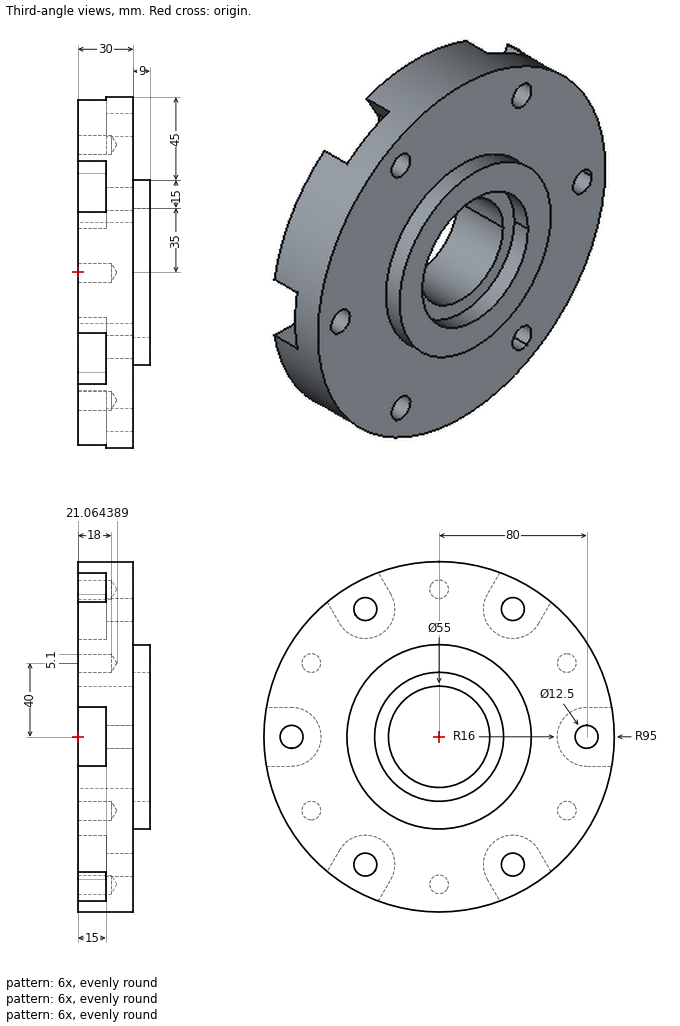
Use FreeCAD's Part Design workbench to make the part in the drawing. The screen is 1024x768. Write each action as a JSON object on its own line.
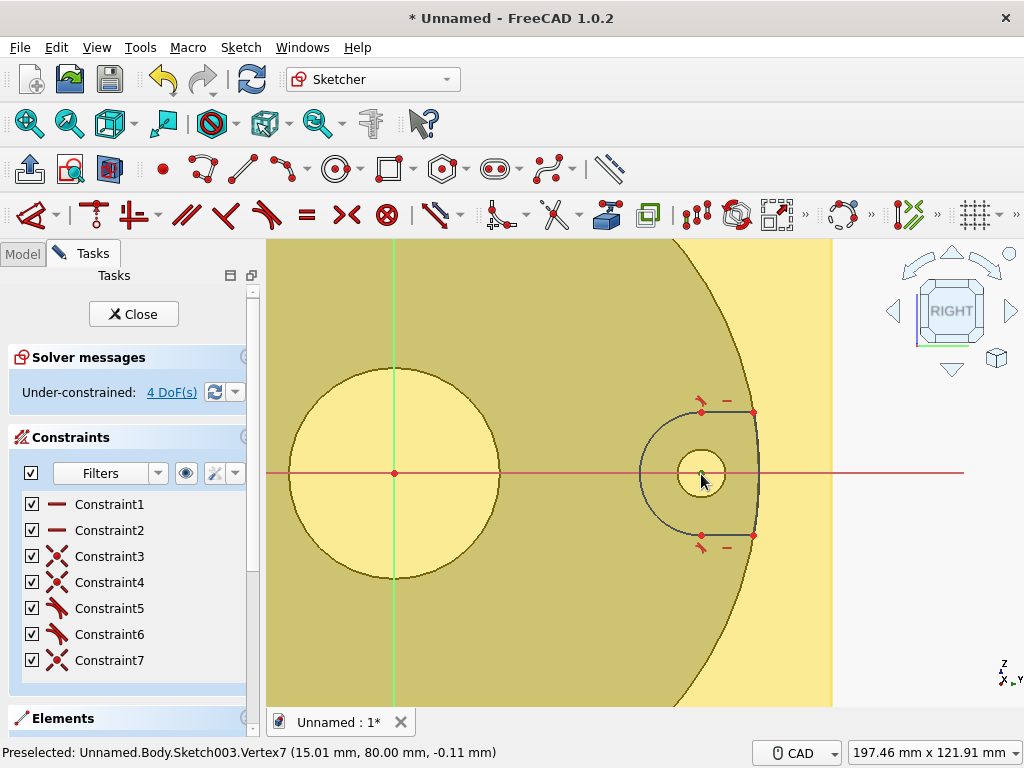
{"action": "left_click", "coordinate": [334, 473]}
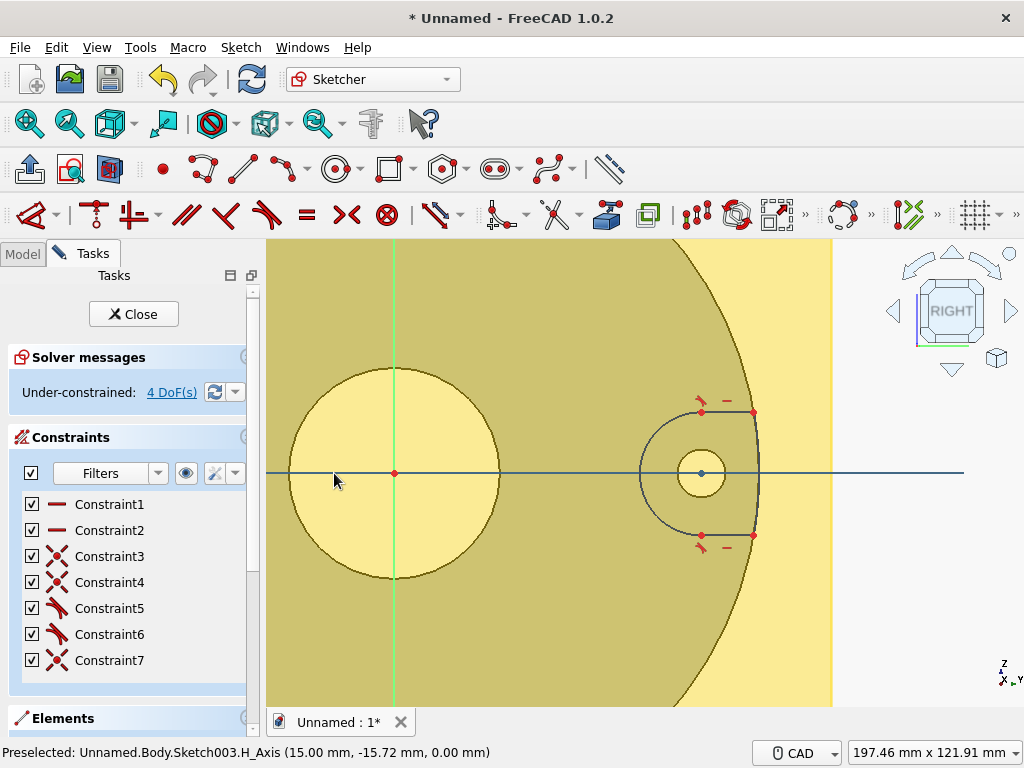
{"action": "key", "text": "c"}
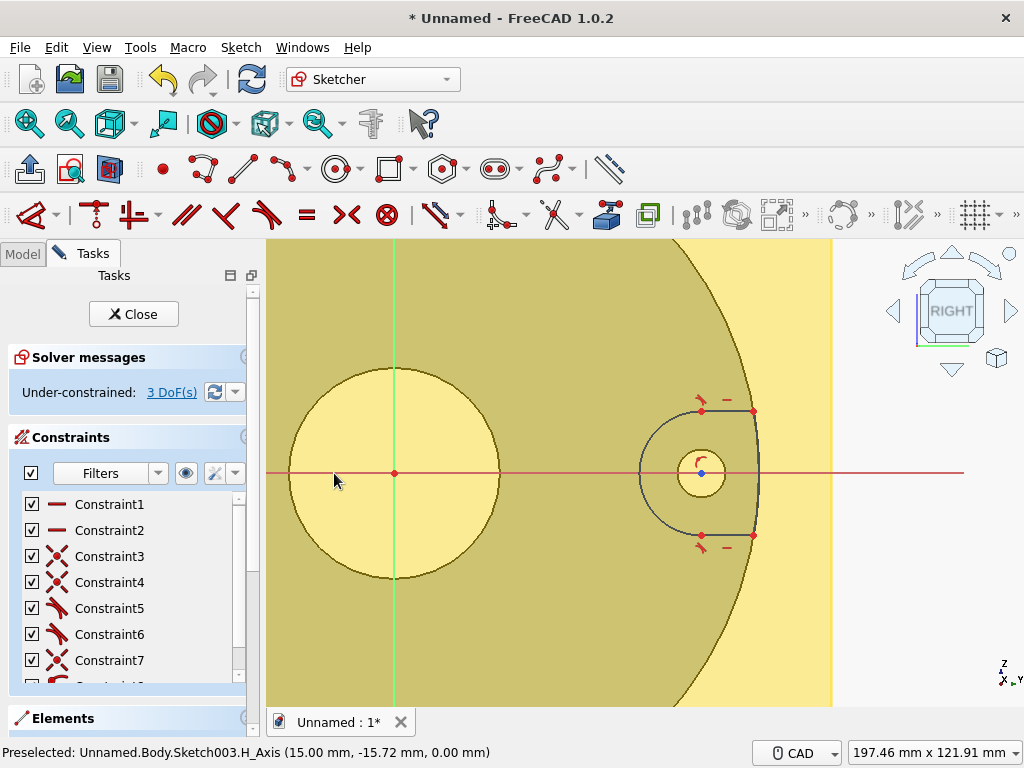
{"action": "left_click", "coordinate": [32, 216]}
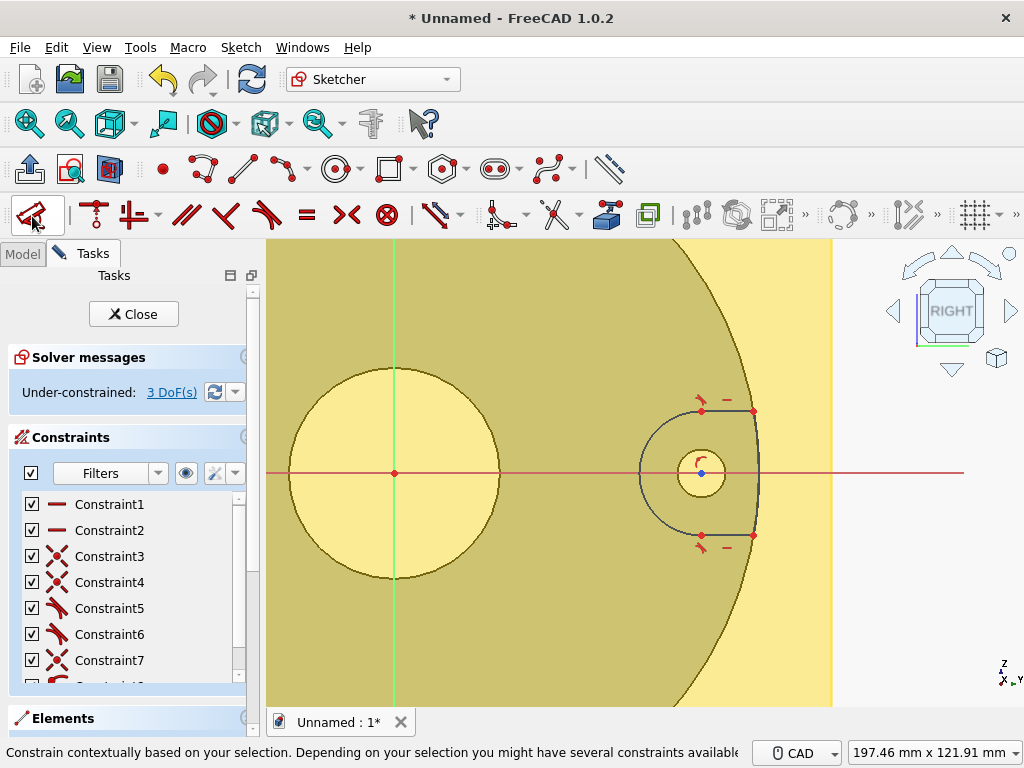
{"action": "left_click", "coordinate": [651, 437]}
{"action": "left_click", "coordinate": [625, 418]}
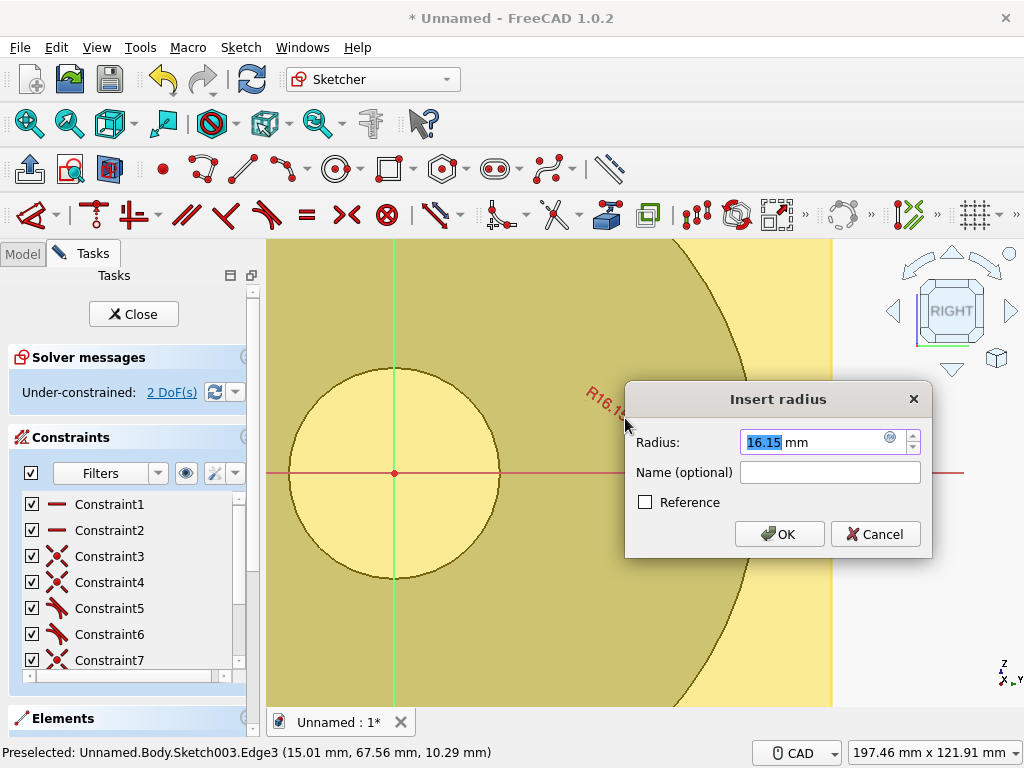
{"action": "type", "text": "16"}
{"action": "key", "text": "Return"}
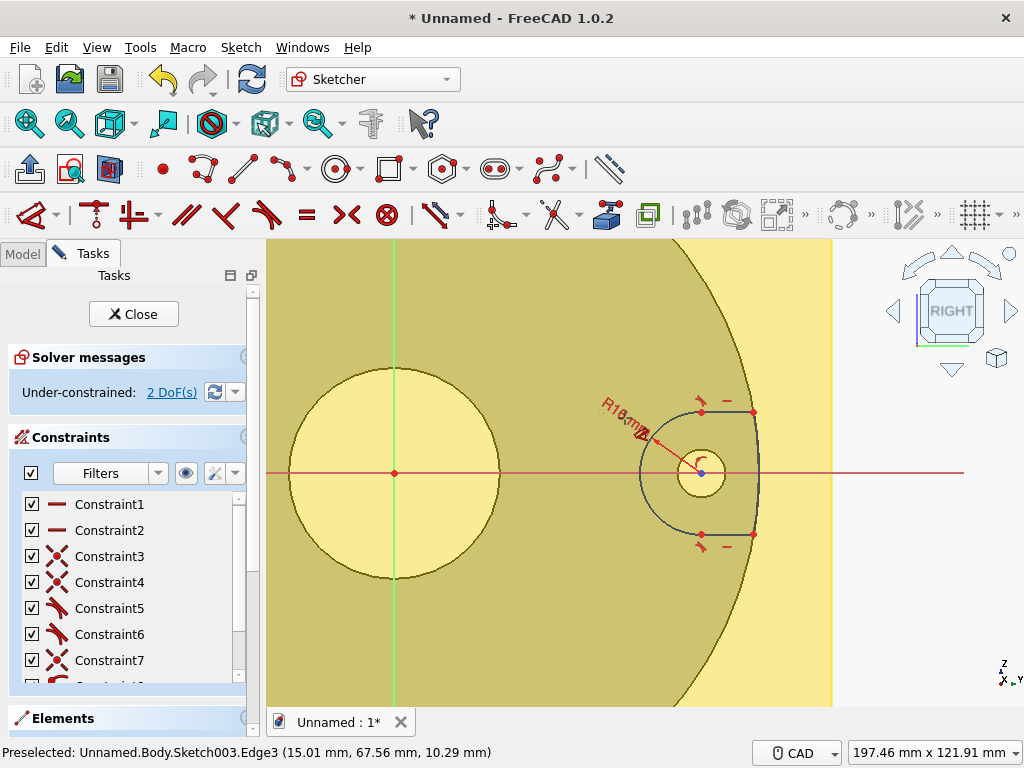
{"action": "left_click", "coordinate": [758, 498]}
{"action": "left_click", "coordinate": [790, 500]}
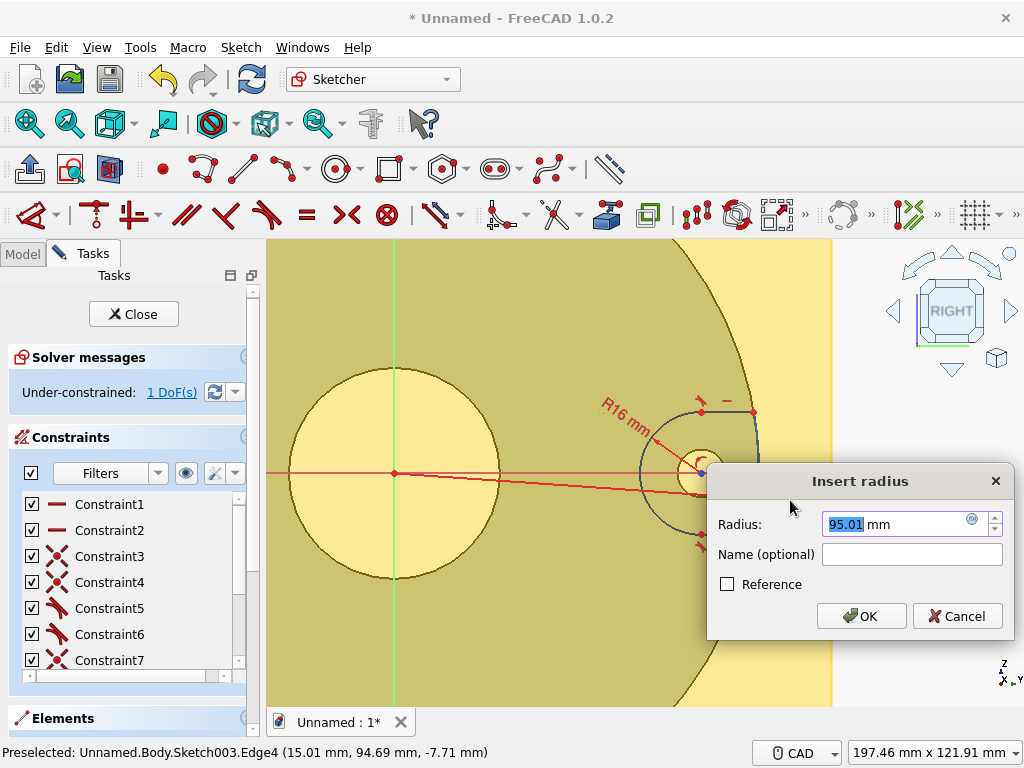
{"action": "type", "text": "95"}
{"action": "key", "text": "Return"}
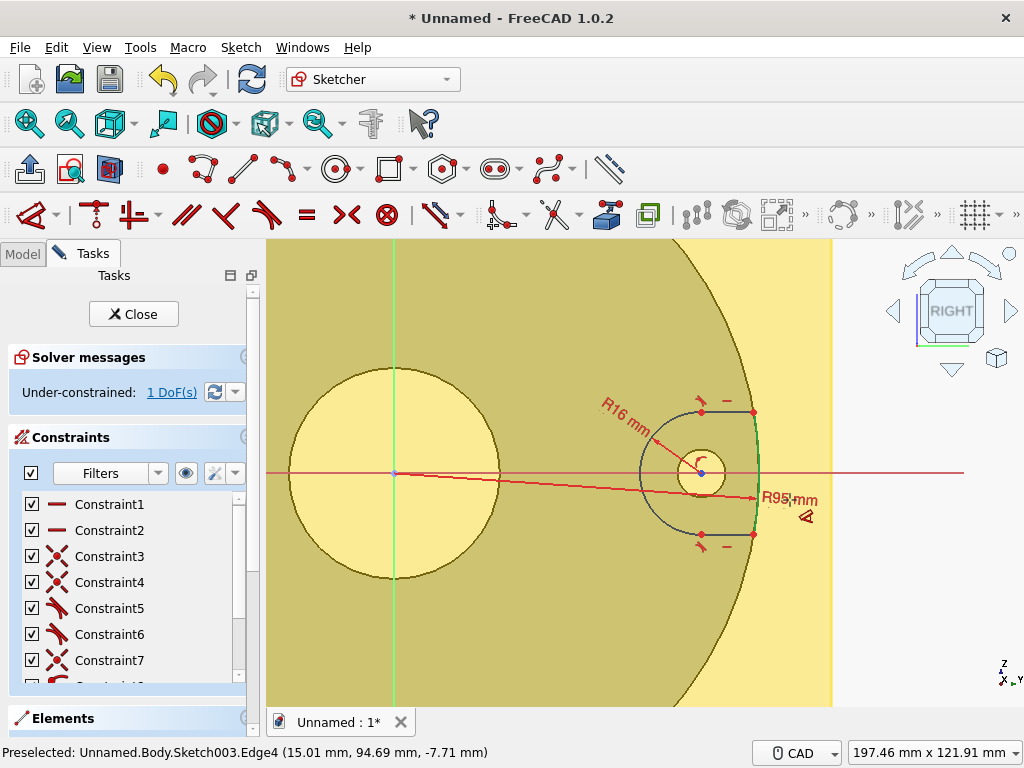
{"action": "left_click", "coordinate": [701, 535]}
{"action": "left_click", "coordinate": [548, 569]}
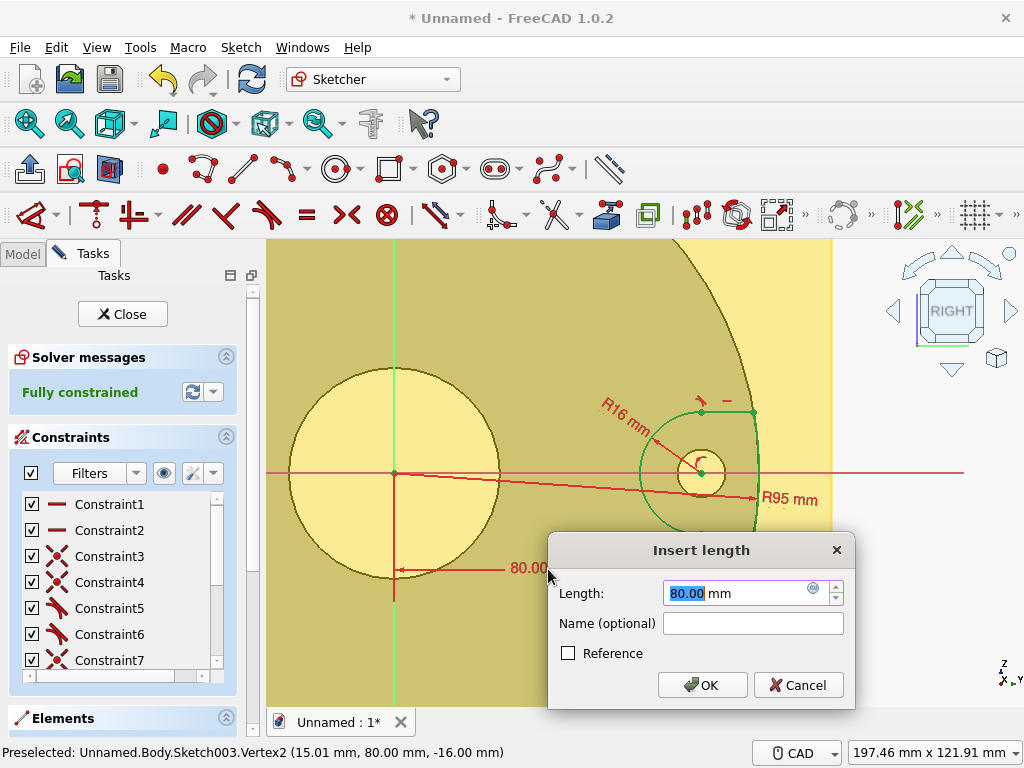
{"action": "type", "text": "80"}
{"action": "key", "text": "Return"}
{"action": "key", "text": "Escape"}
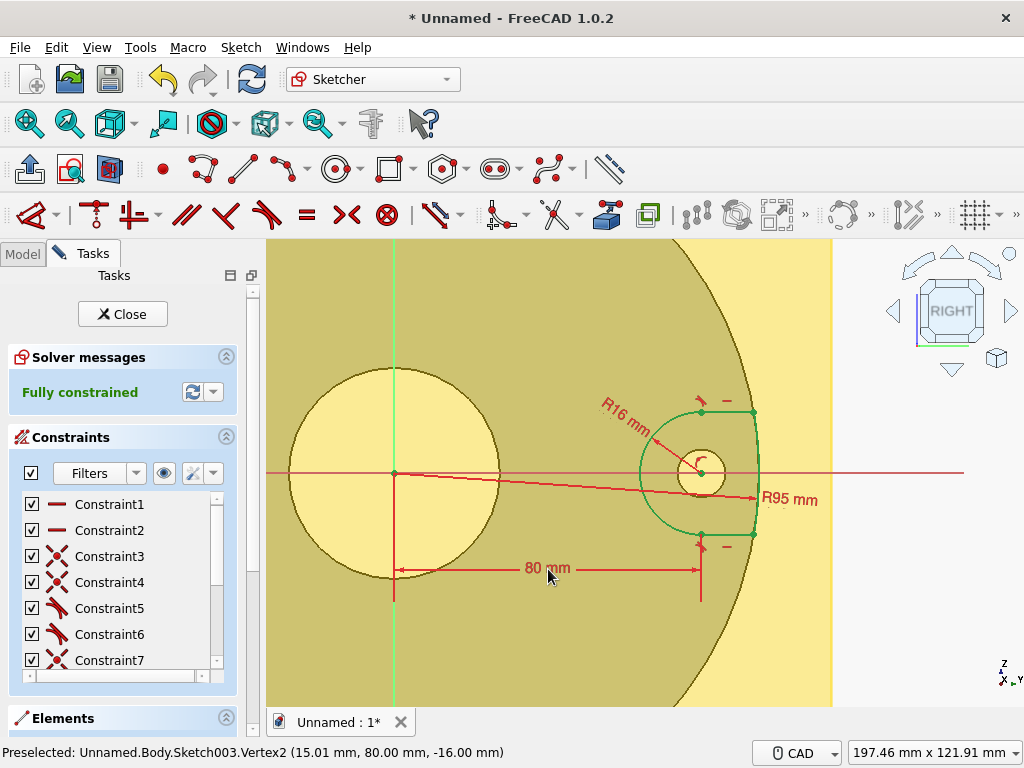
{"action": "left_click", "coordinate": [123, 314]}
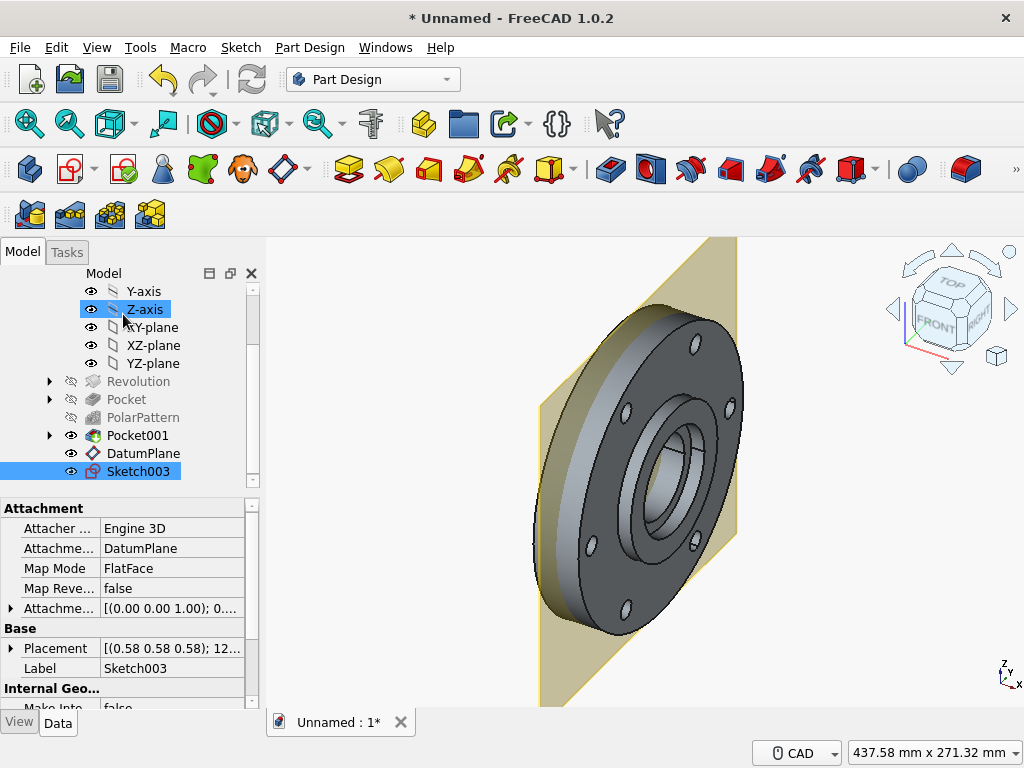
{"action": "left_click", "coordinate": [612, 170]}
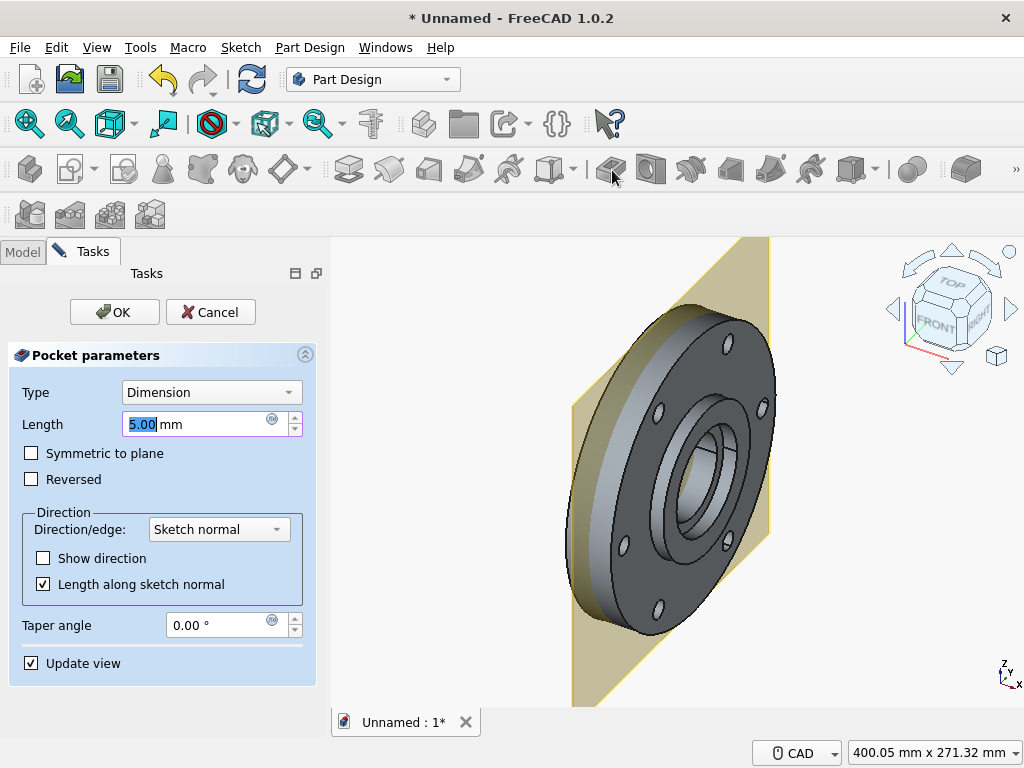
{"action": "type", "text": "15"}
{"action": "key", "text": "Tab"}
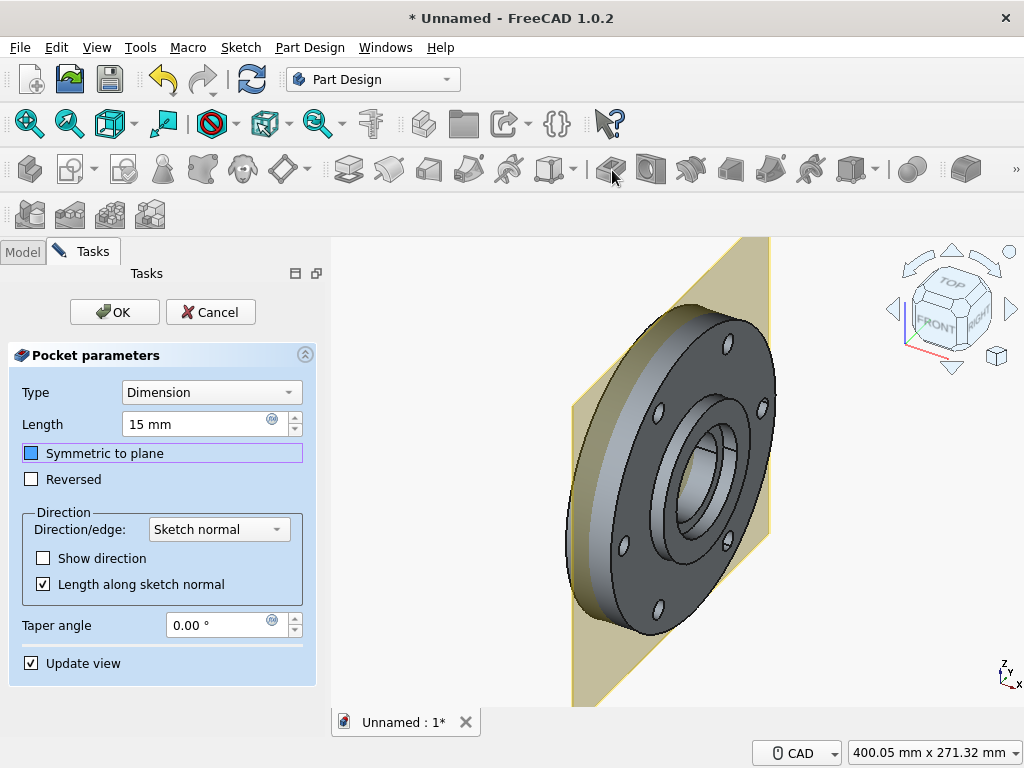
{"action": "left_click", "coordinate": [115, 312]}